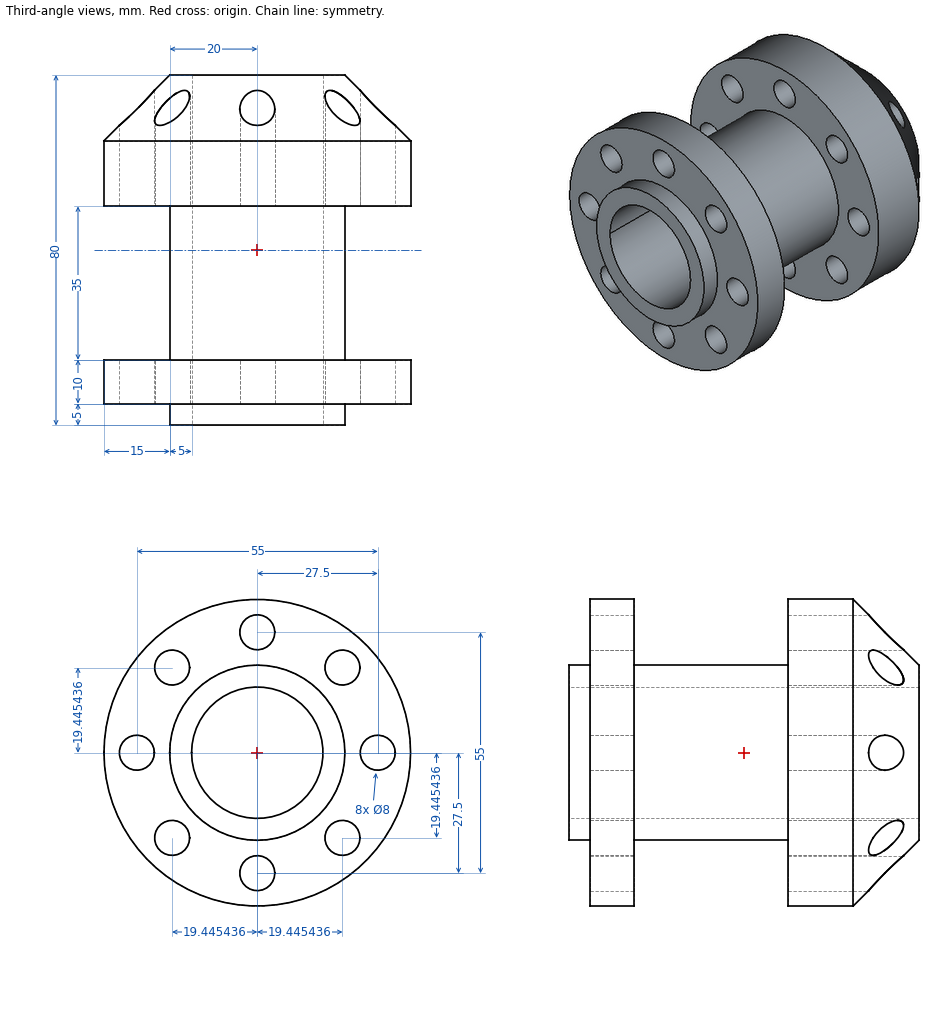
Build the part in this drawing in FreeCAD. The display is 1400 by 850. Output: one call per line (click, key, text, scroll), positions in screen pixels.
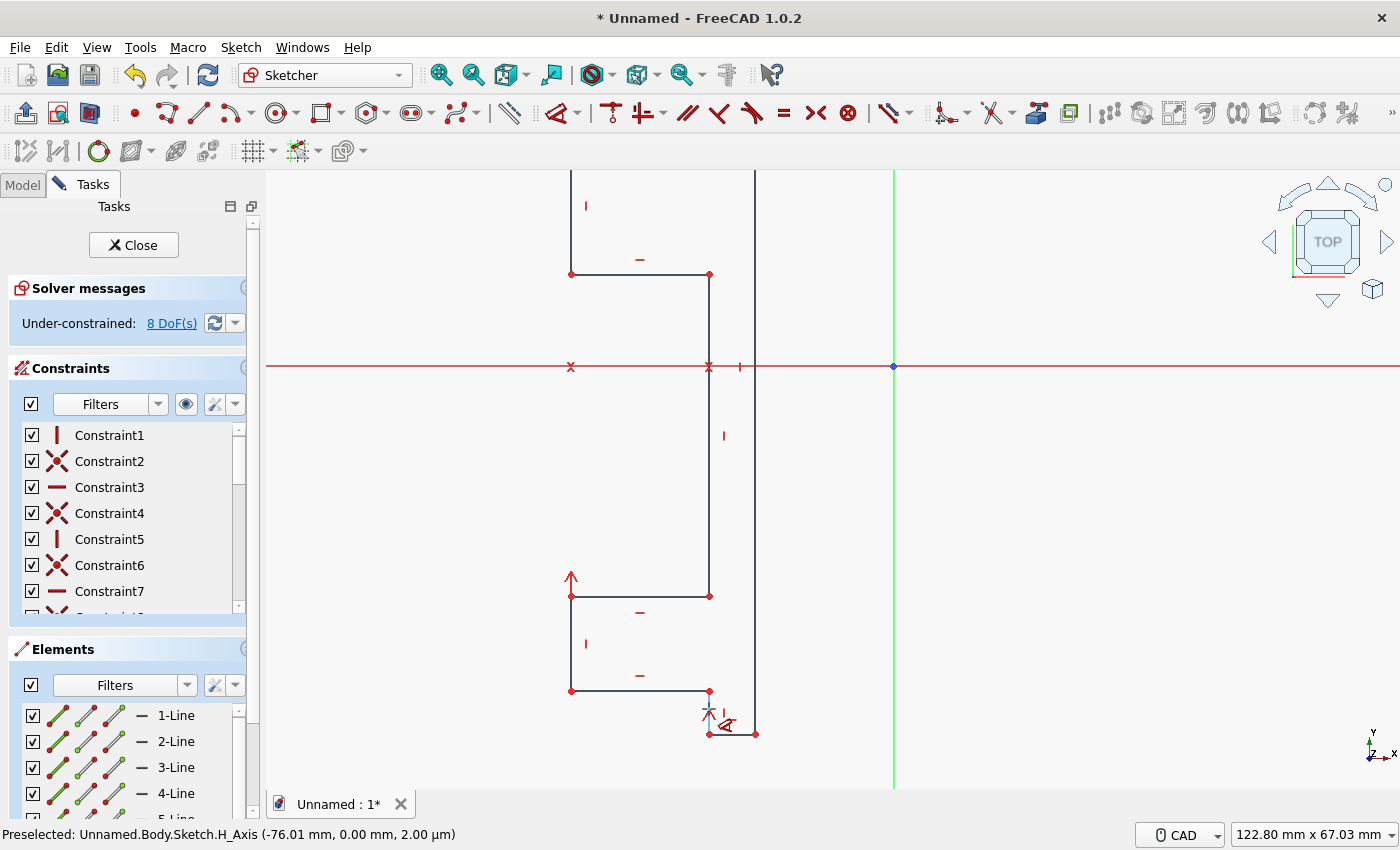
click(709, 709)
click(675, 713)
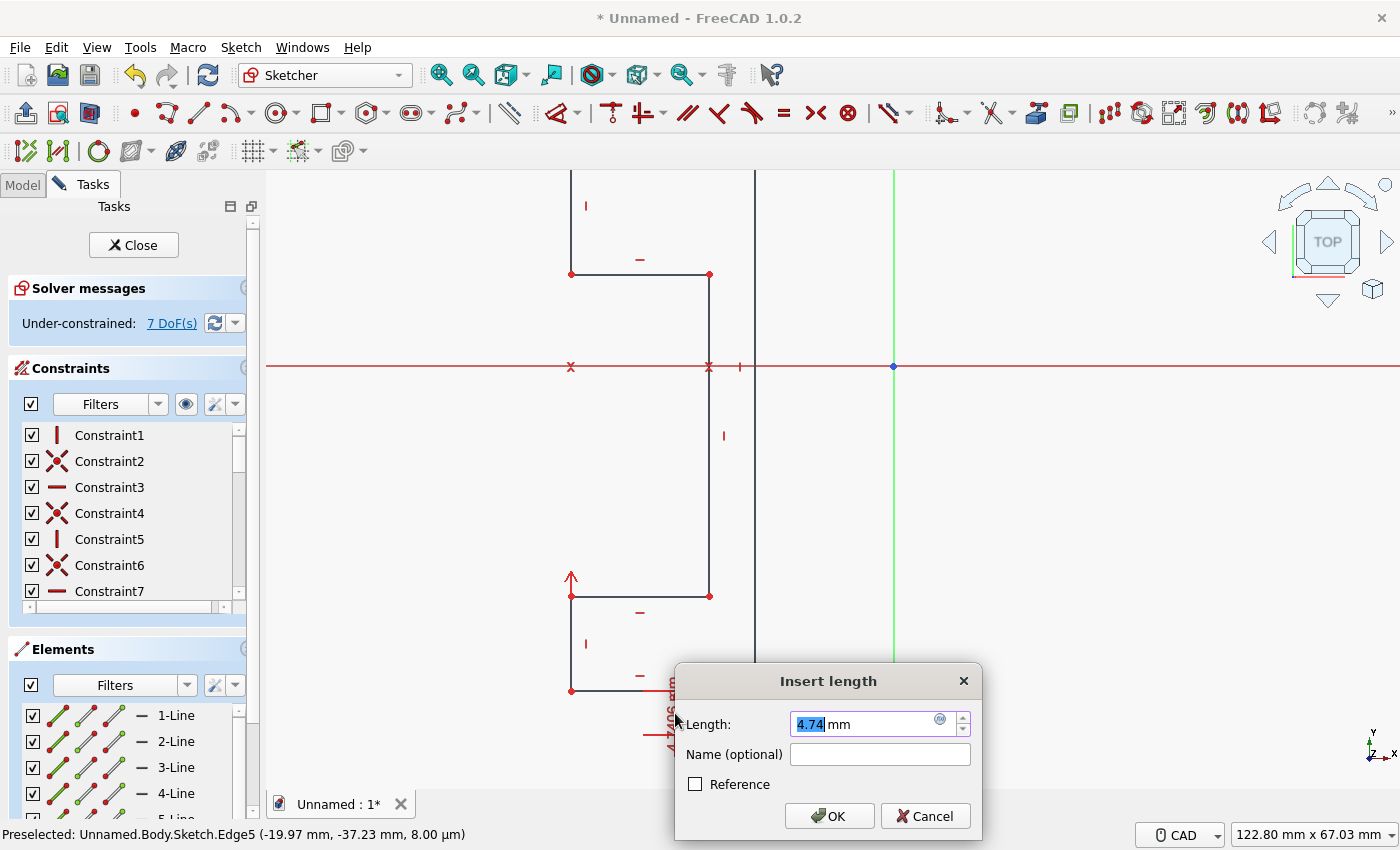
text(5)
key(Return)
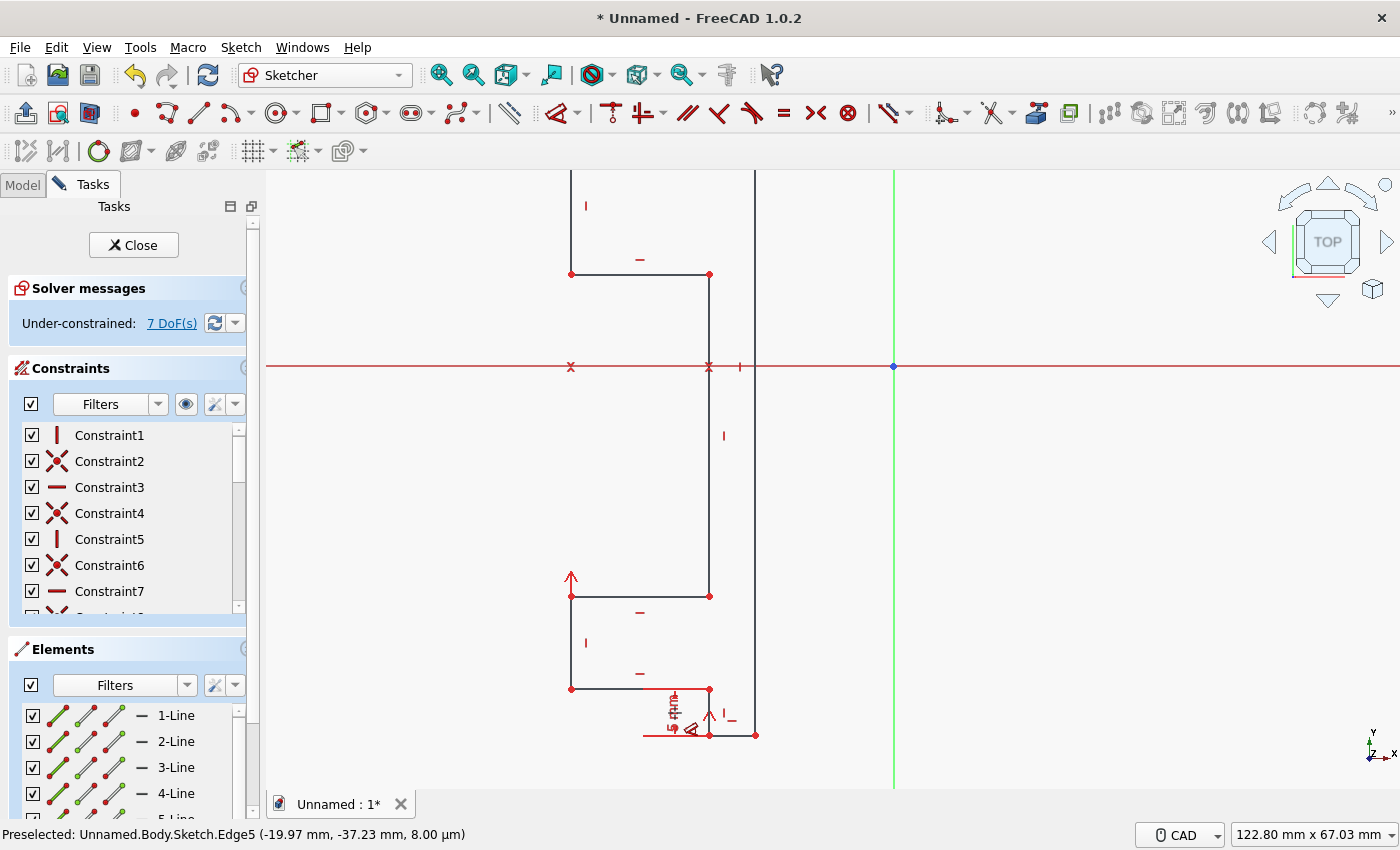
click(723, 736)
click(732, 678)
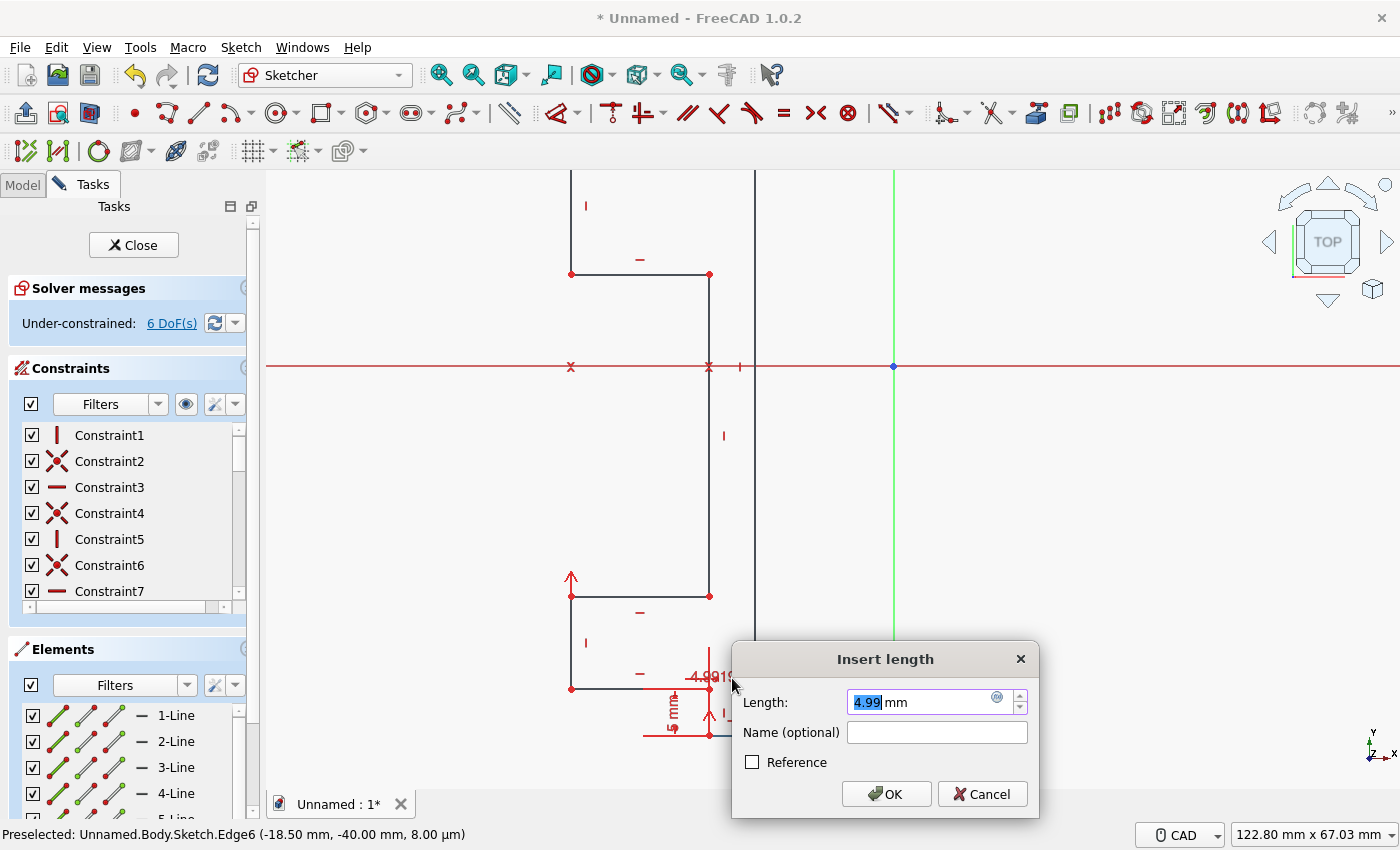
text(5)
key(Return)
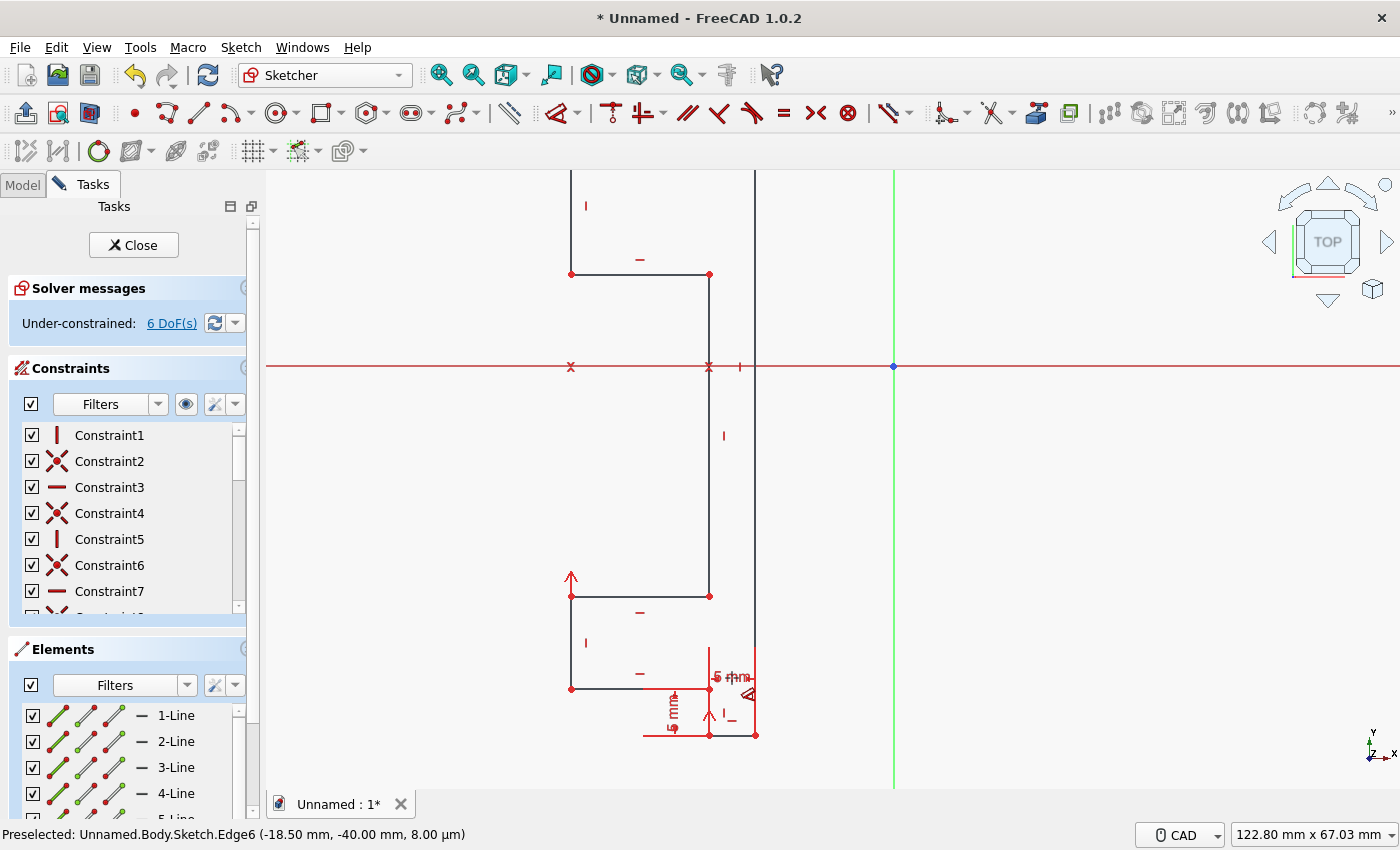
click(709, 500)
click(675, 436)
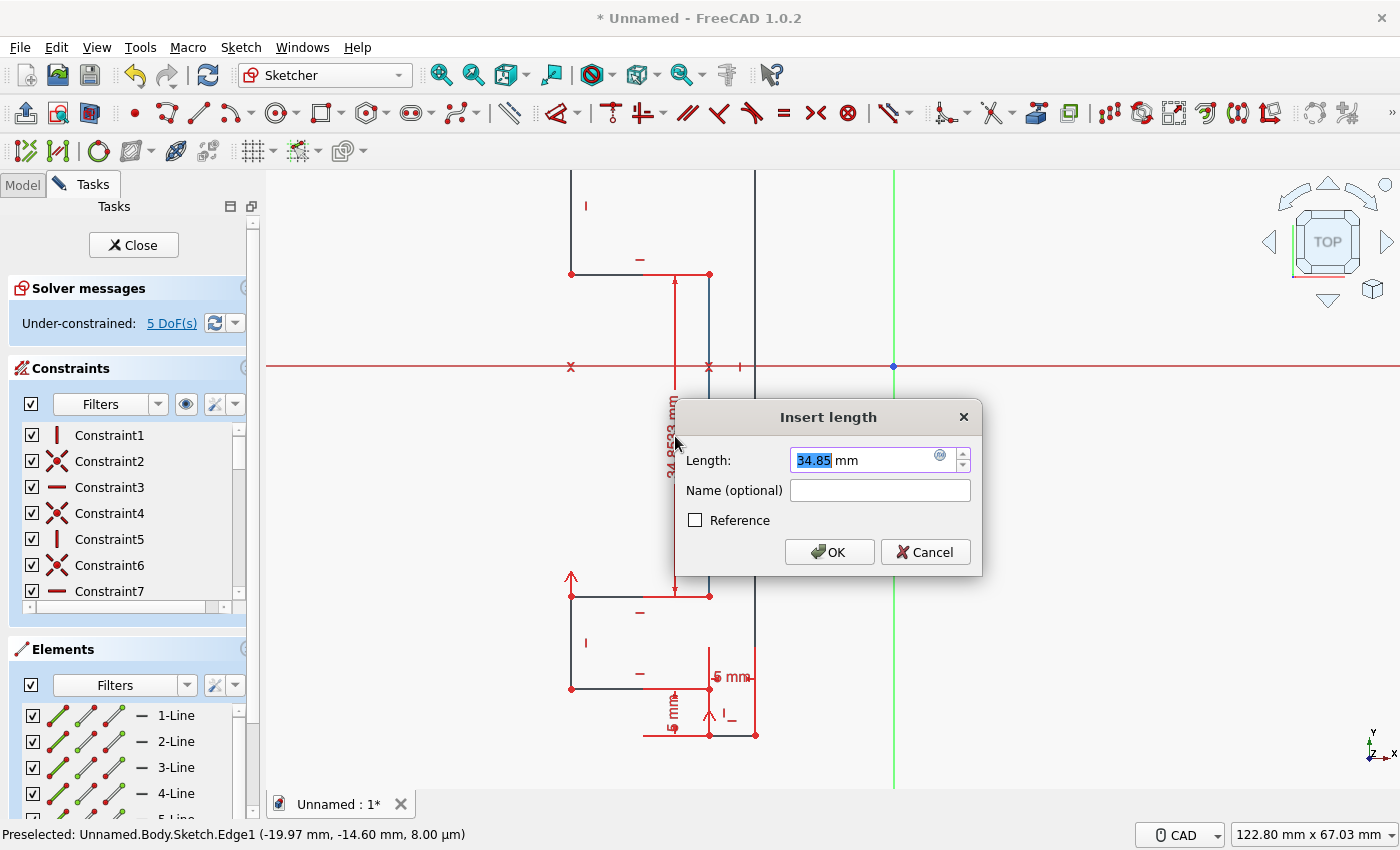
text(35)
key(Return)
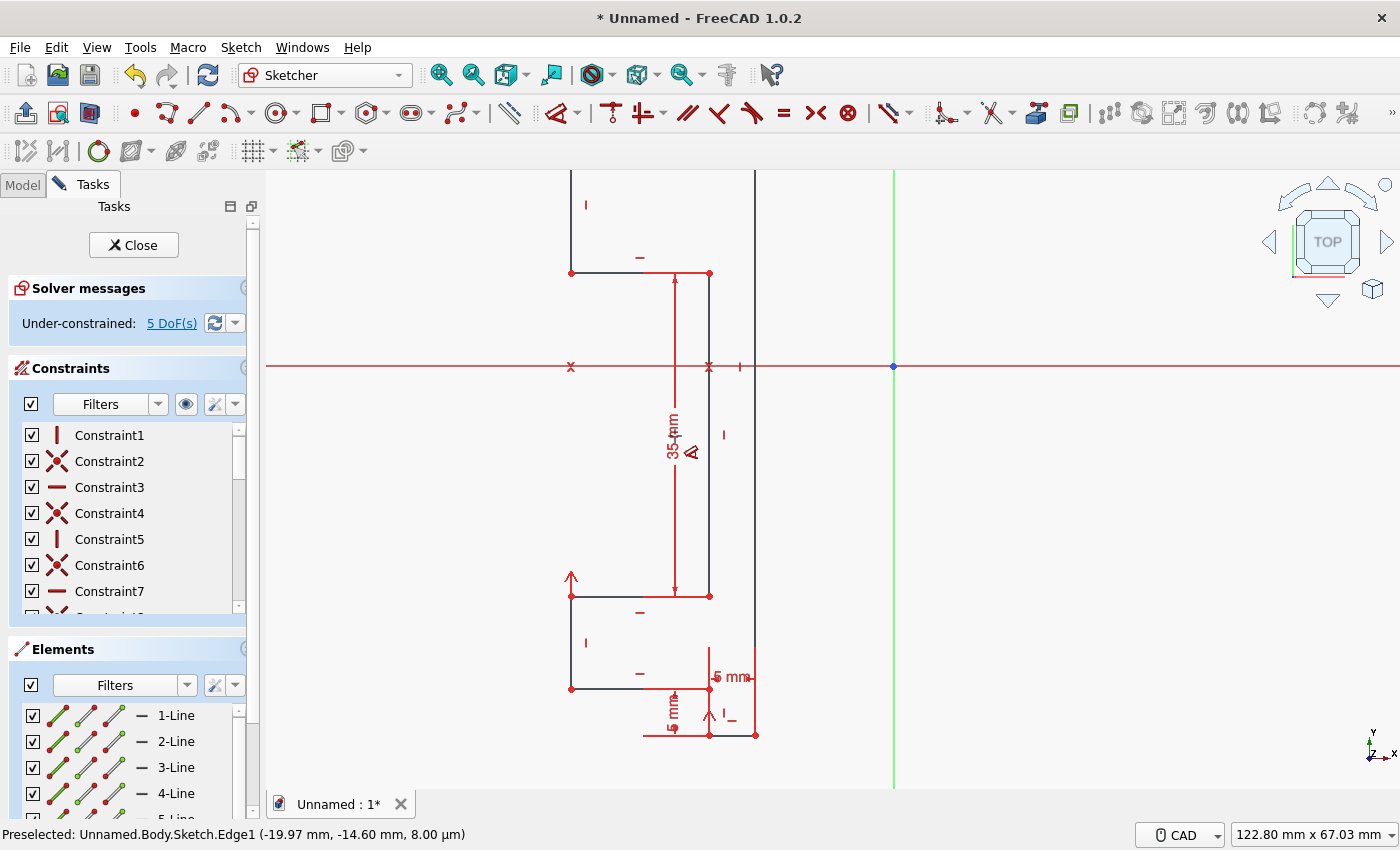
click(668, 597)
click(640, 631)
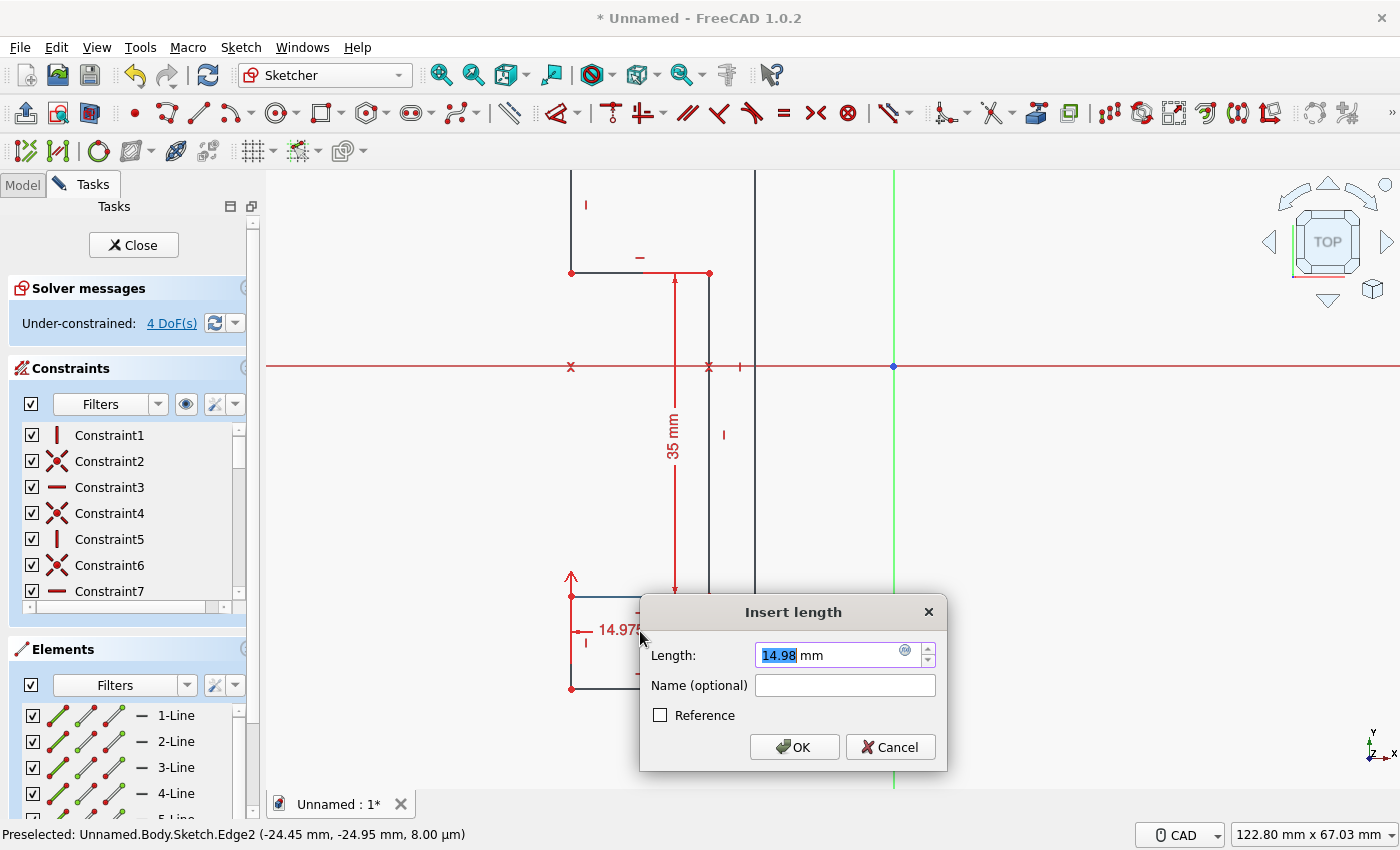
text(15)
key(Return)